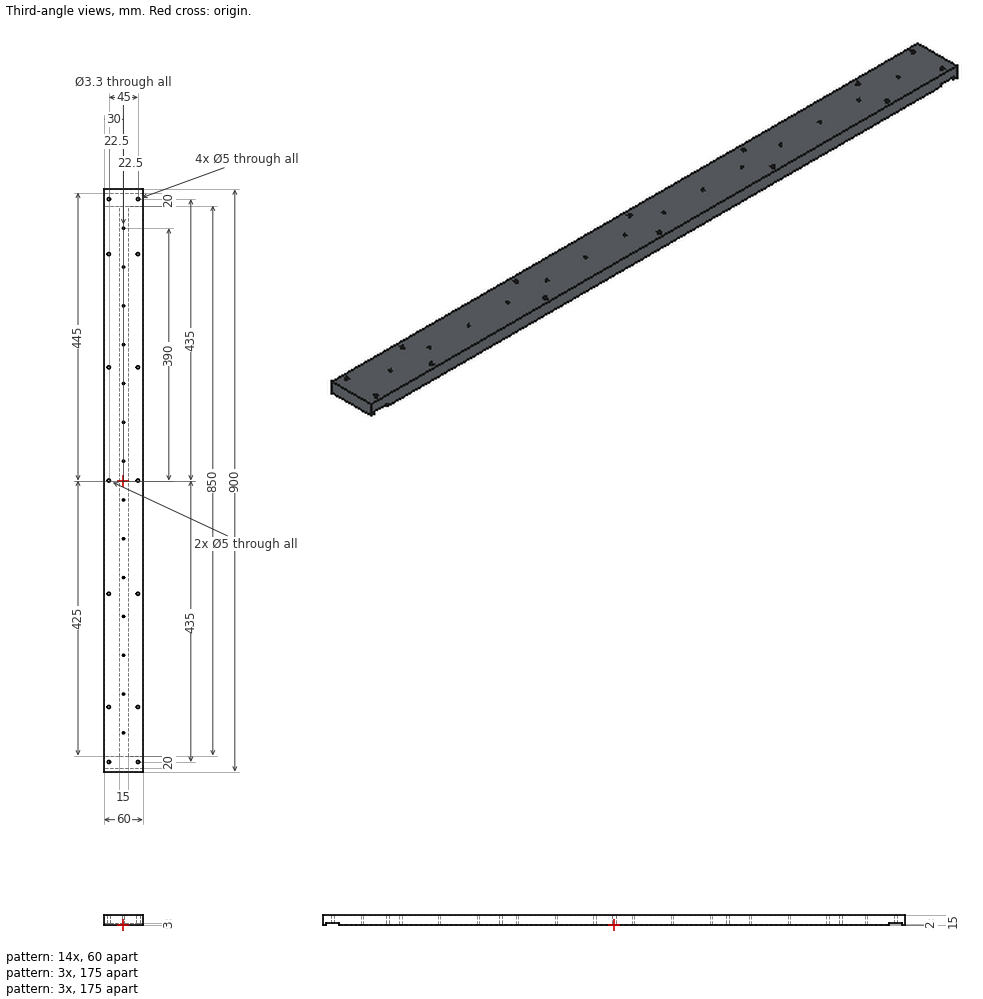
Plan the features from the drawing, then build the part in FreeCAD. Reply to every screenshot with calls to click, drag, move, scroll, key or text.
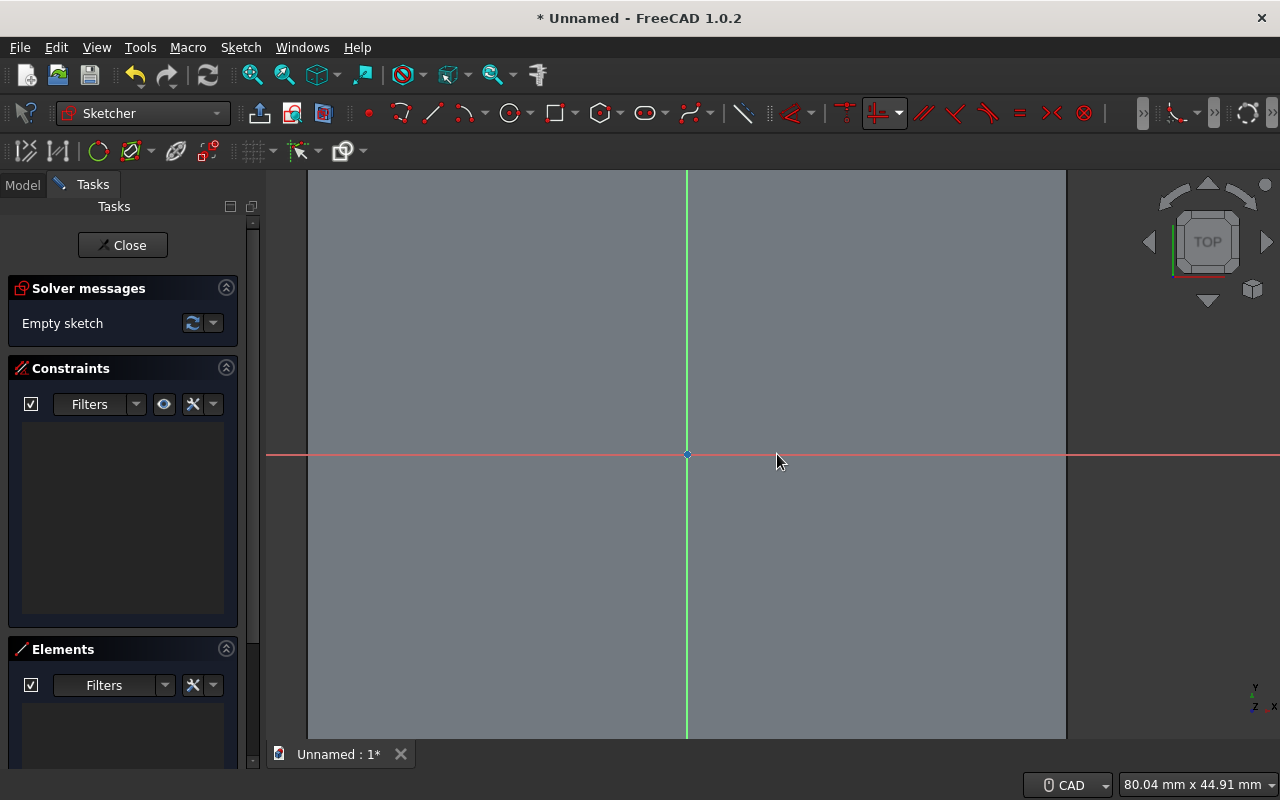
key(g)
key(c)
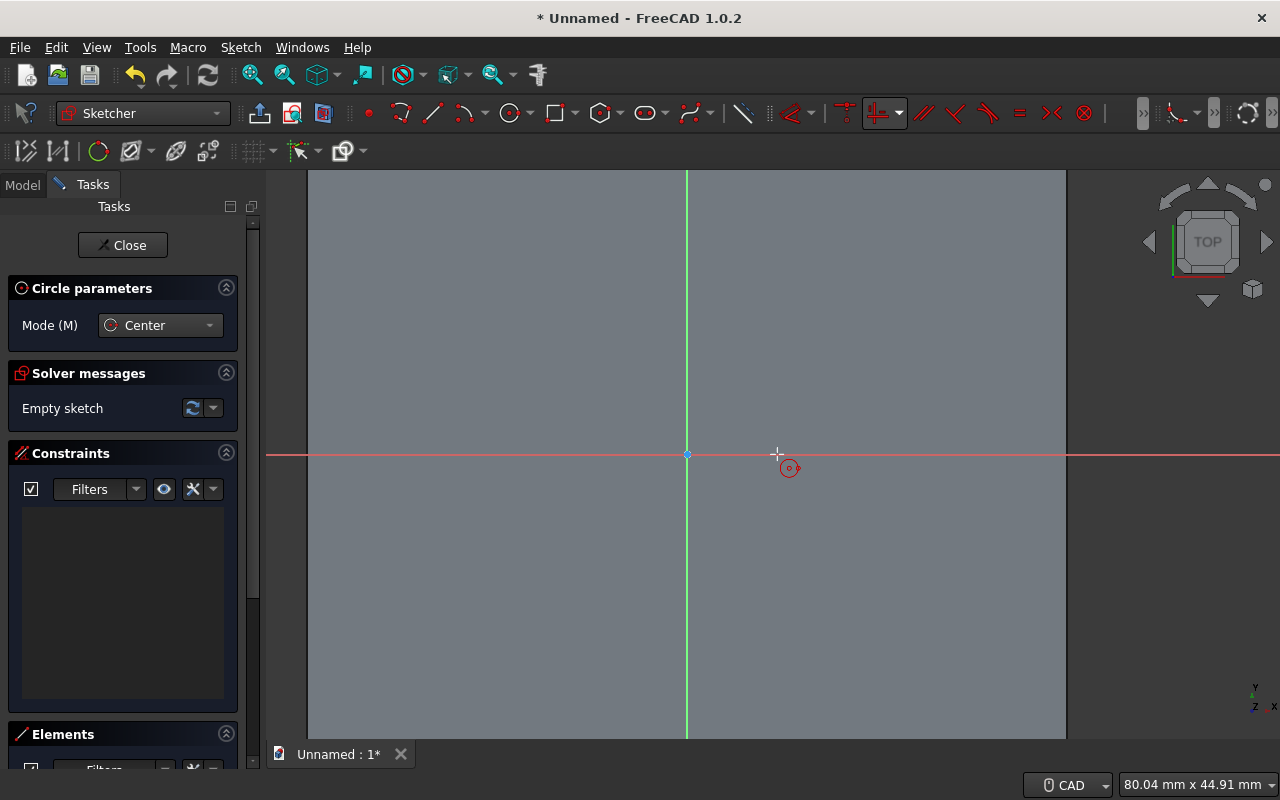
click(402, 454)
move(424, 432)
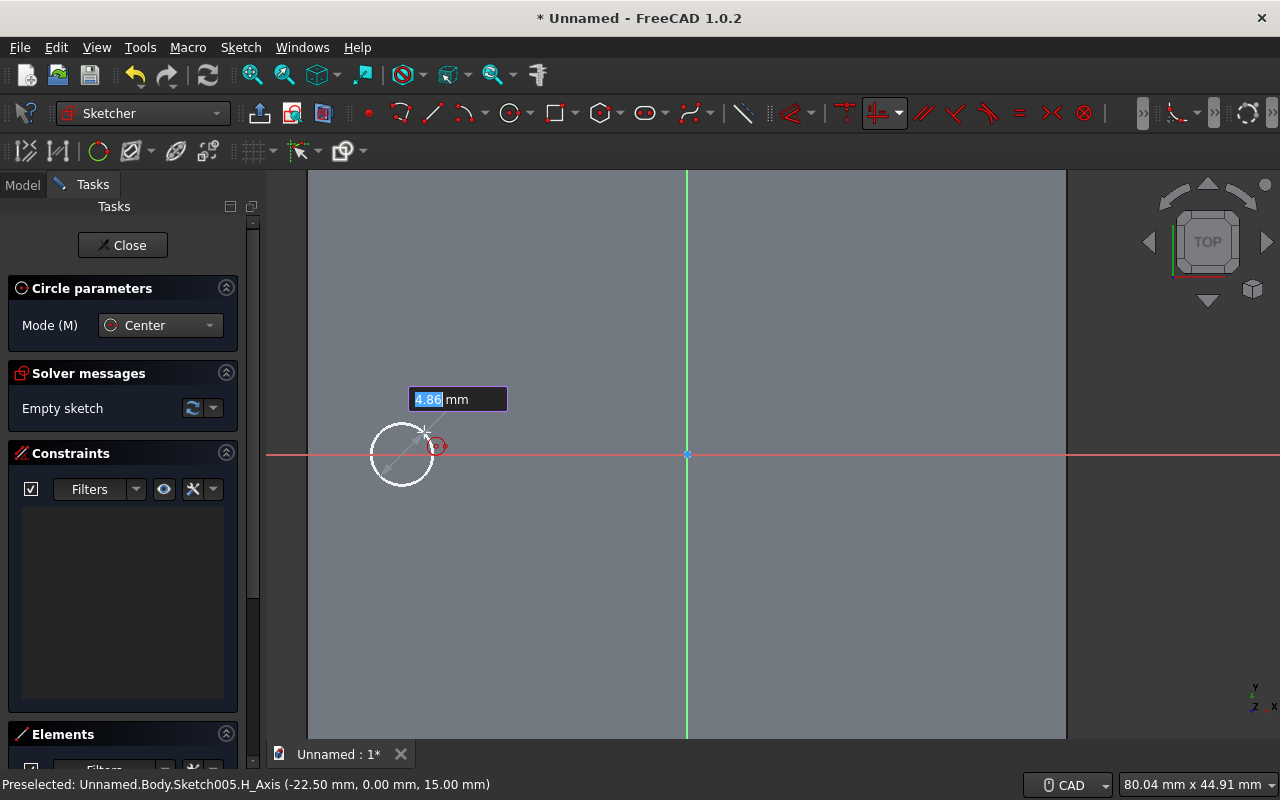
text(5)
key(Return)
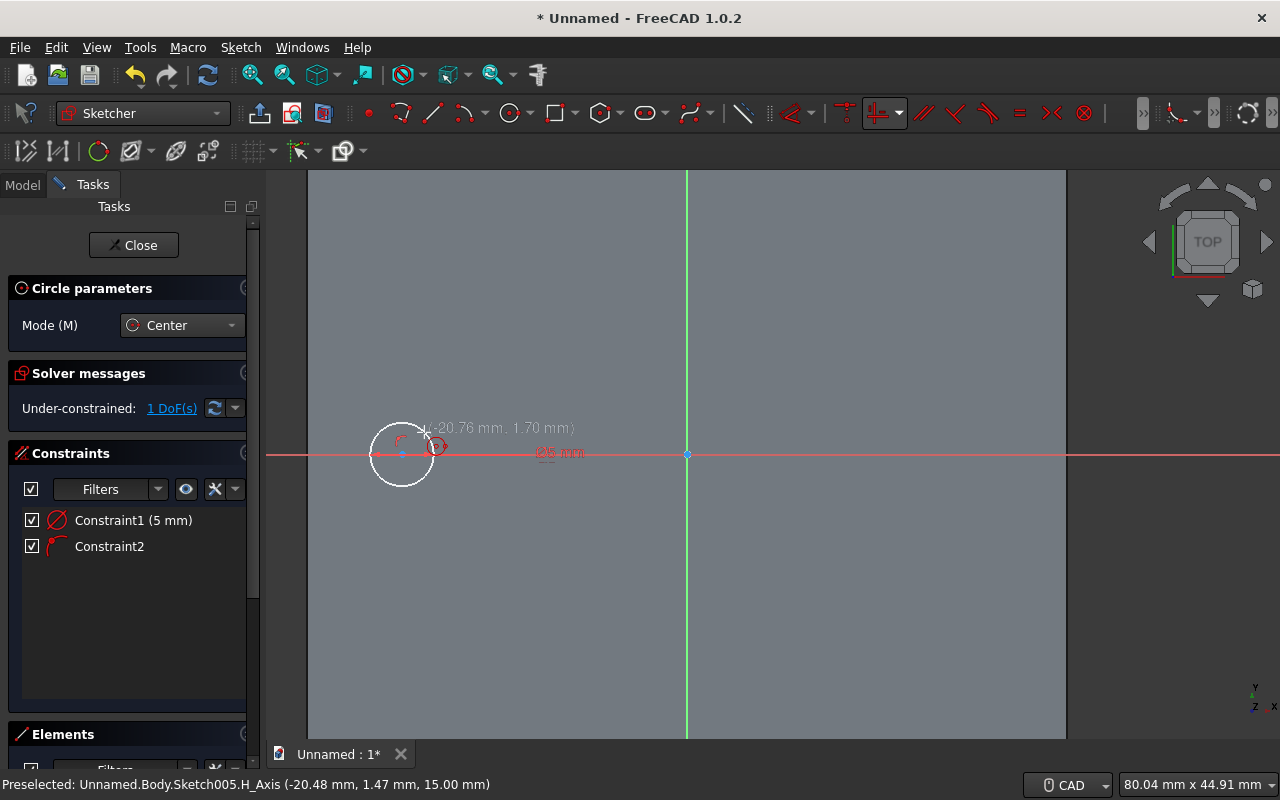
click(972, 454)
move(994, 432)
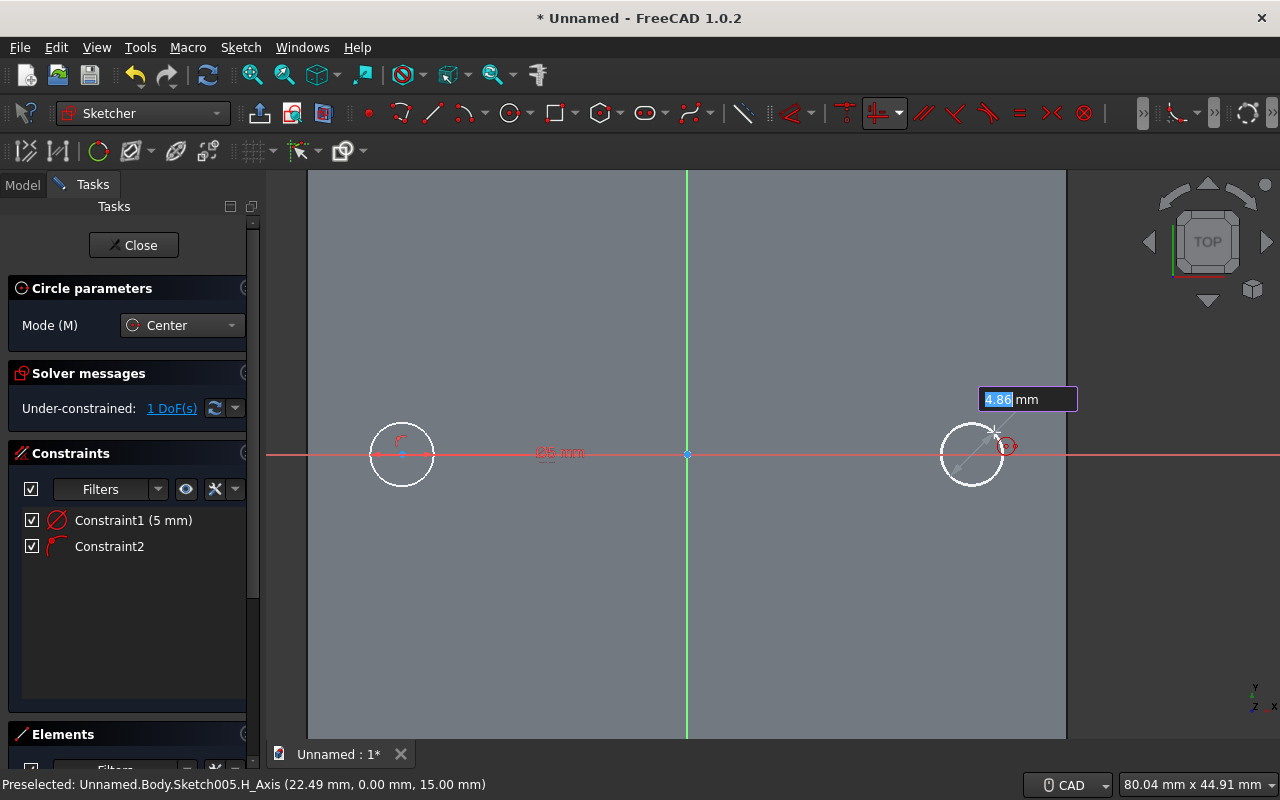
text(5)
key(Return)
key(Escape)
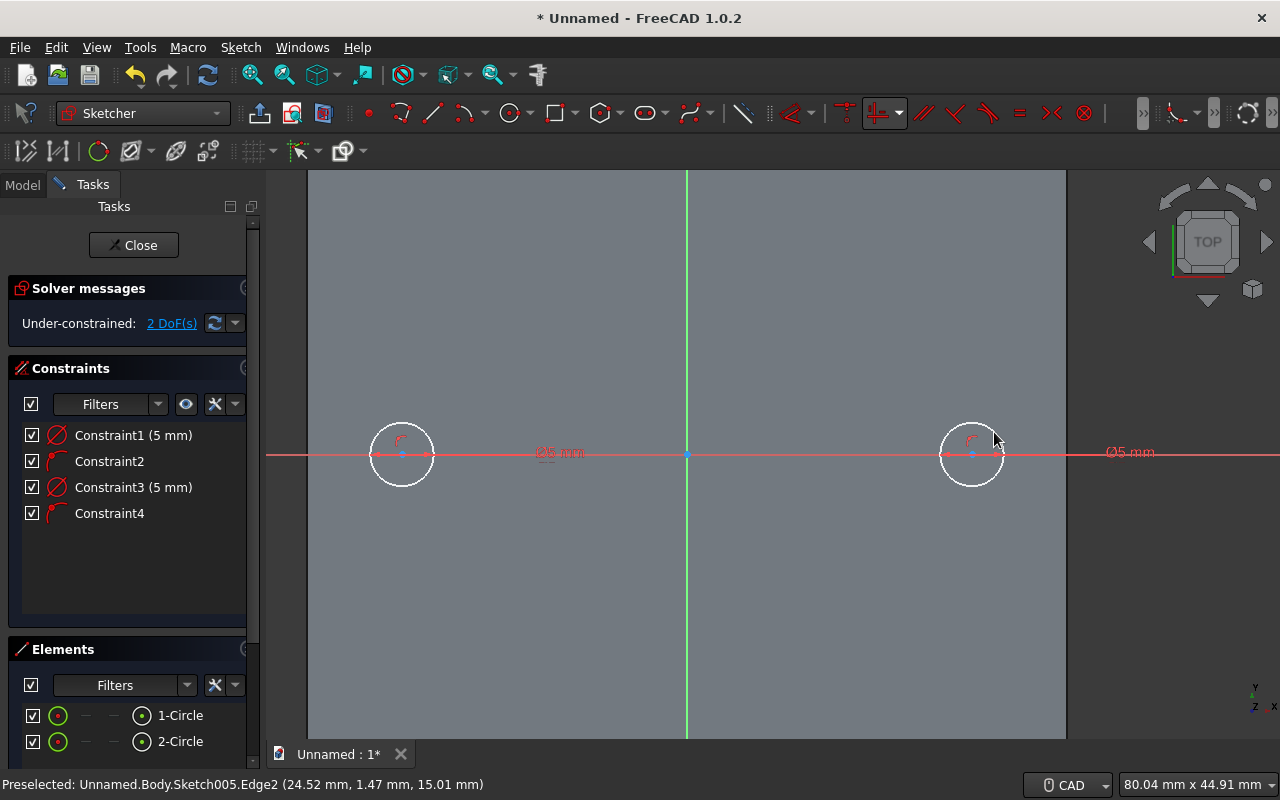
click(790, 114)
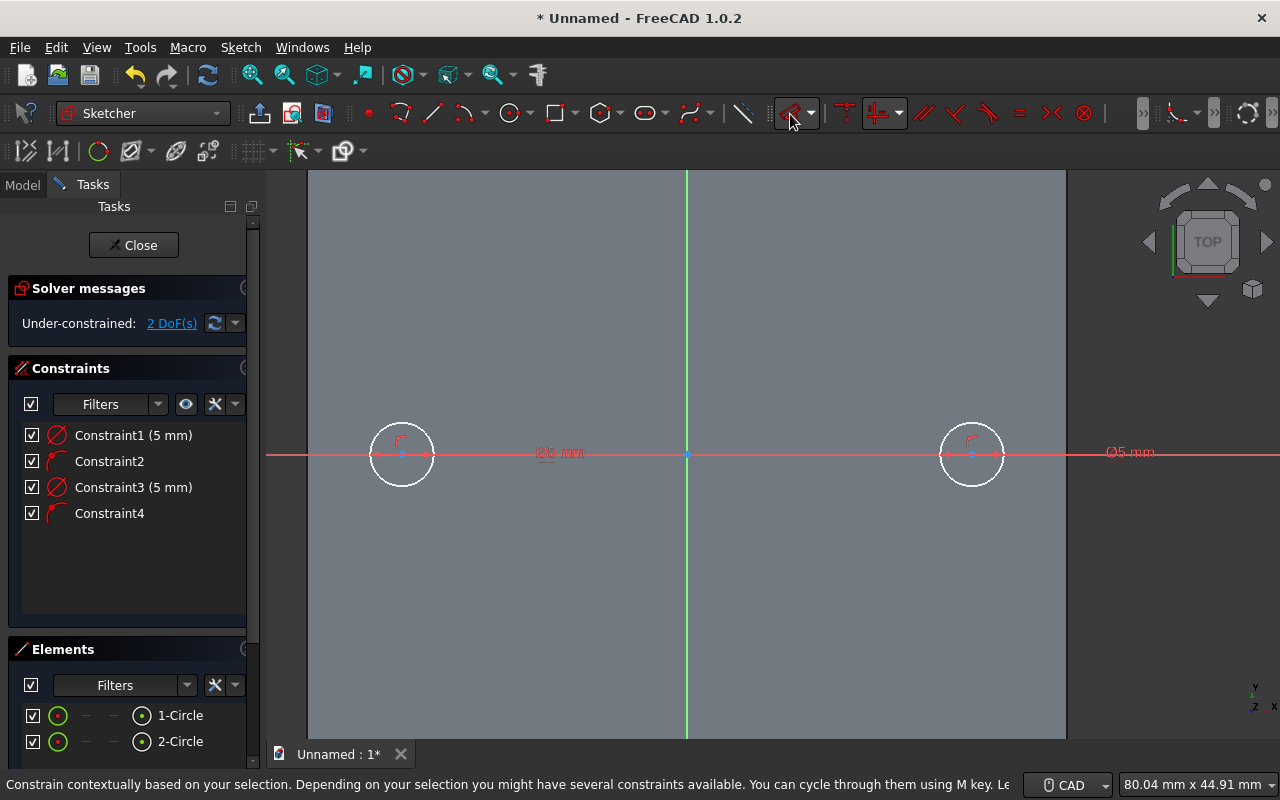
click(402, 454)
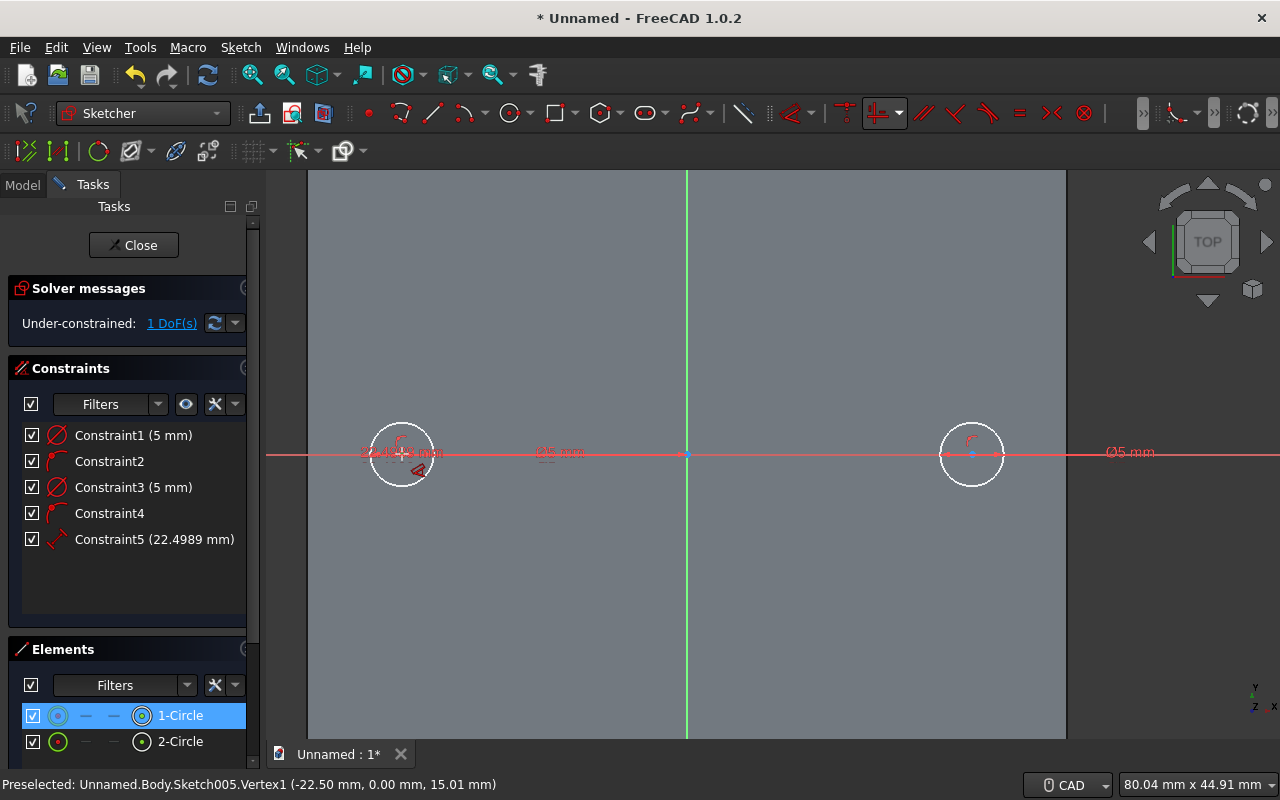
click(972, 454)
click(556, 488)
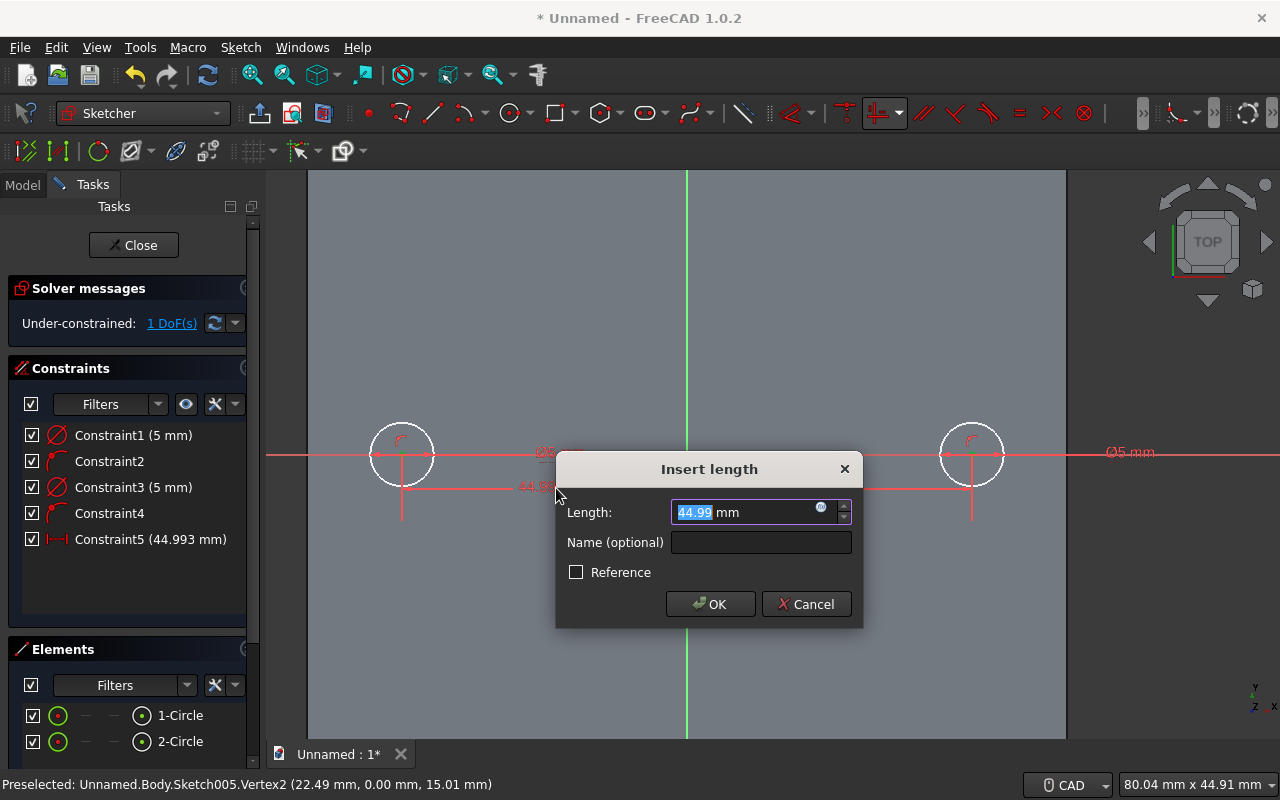
text(45)
key(Return)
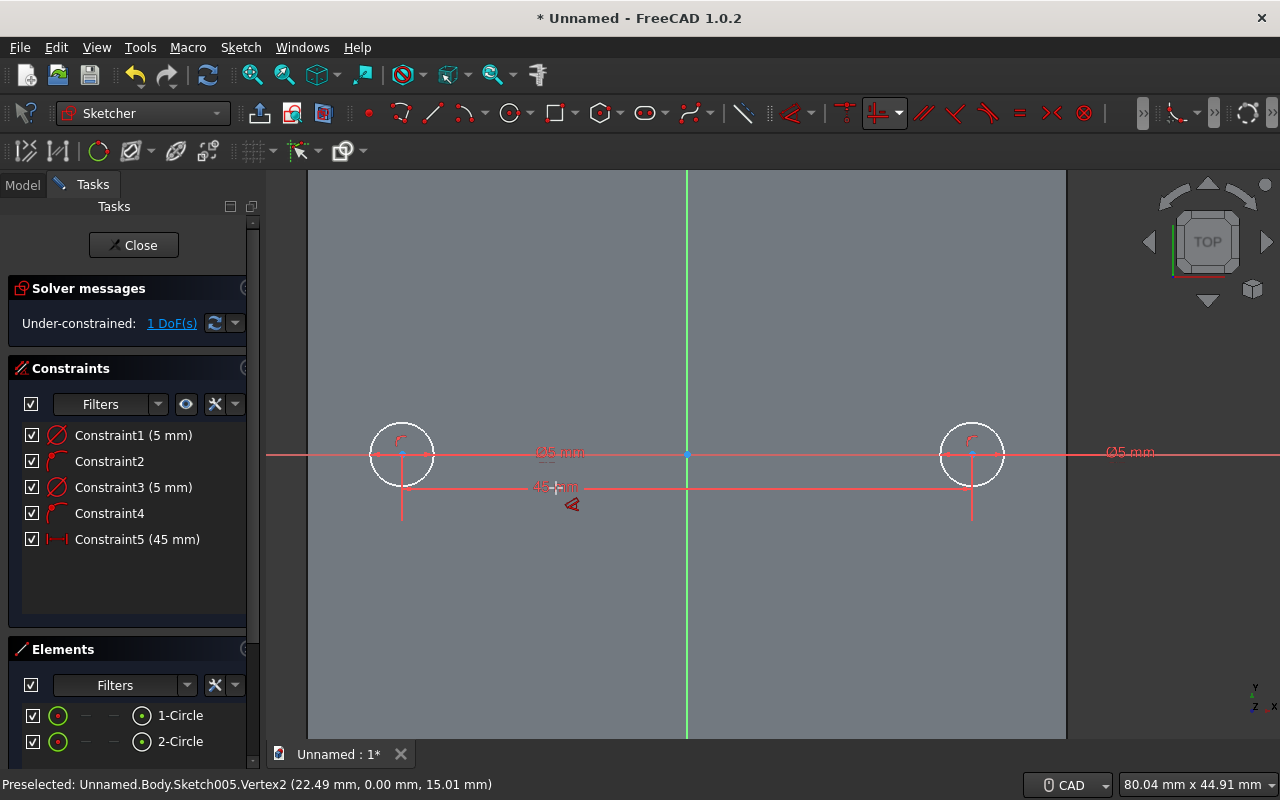
click(402, 454)
click(479, 488)